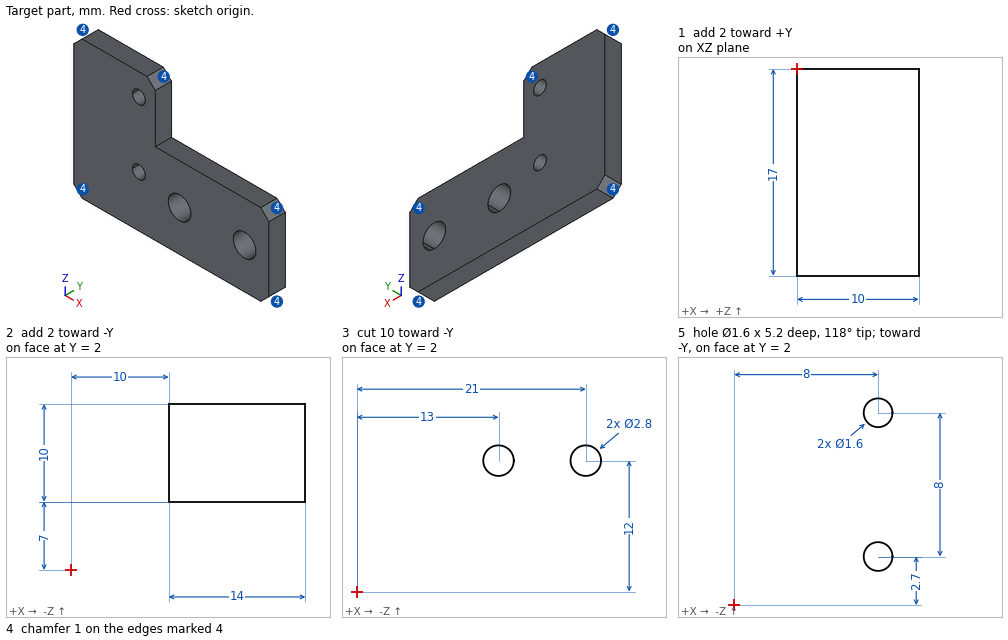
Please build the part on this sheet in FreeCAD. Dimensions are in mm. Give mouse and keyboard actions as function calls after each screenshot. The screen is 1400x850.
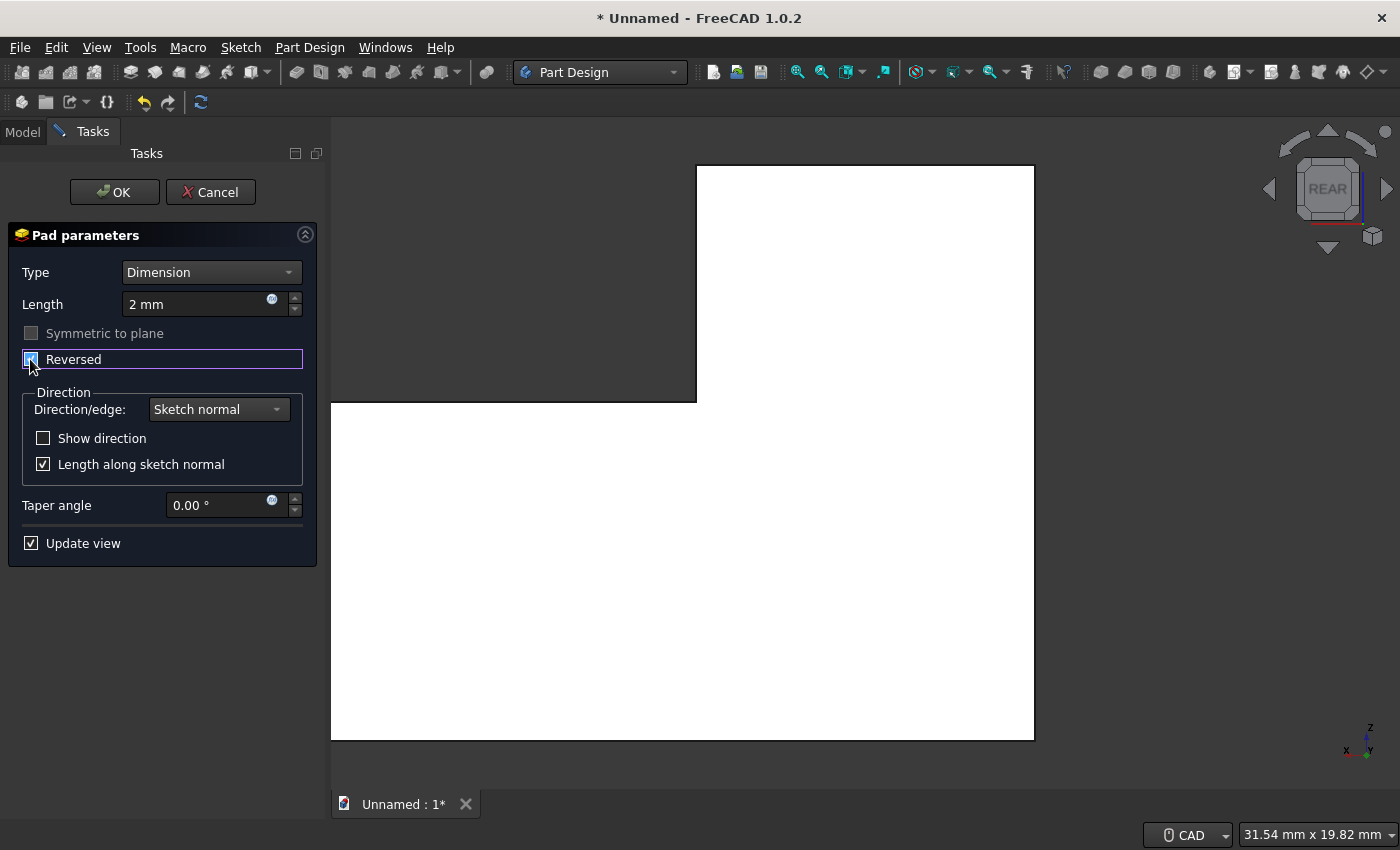
click(115, 192)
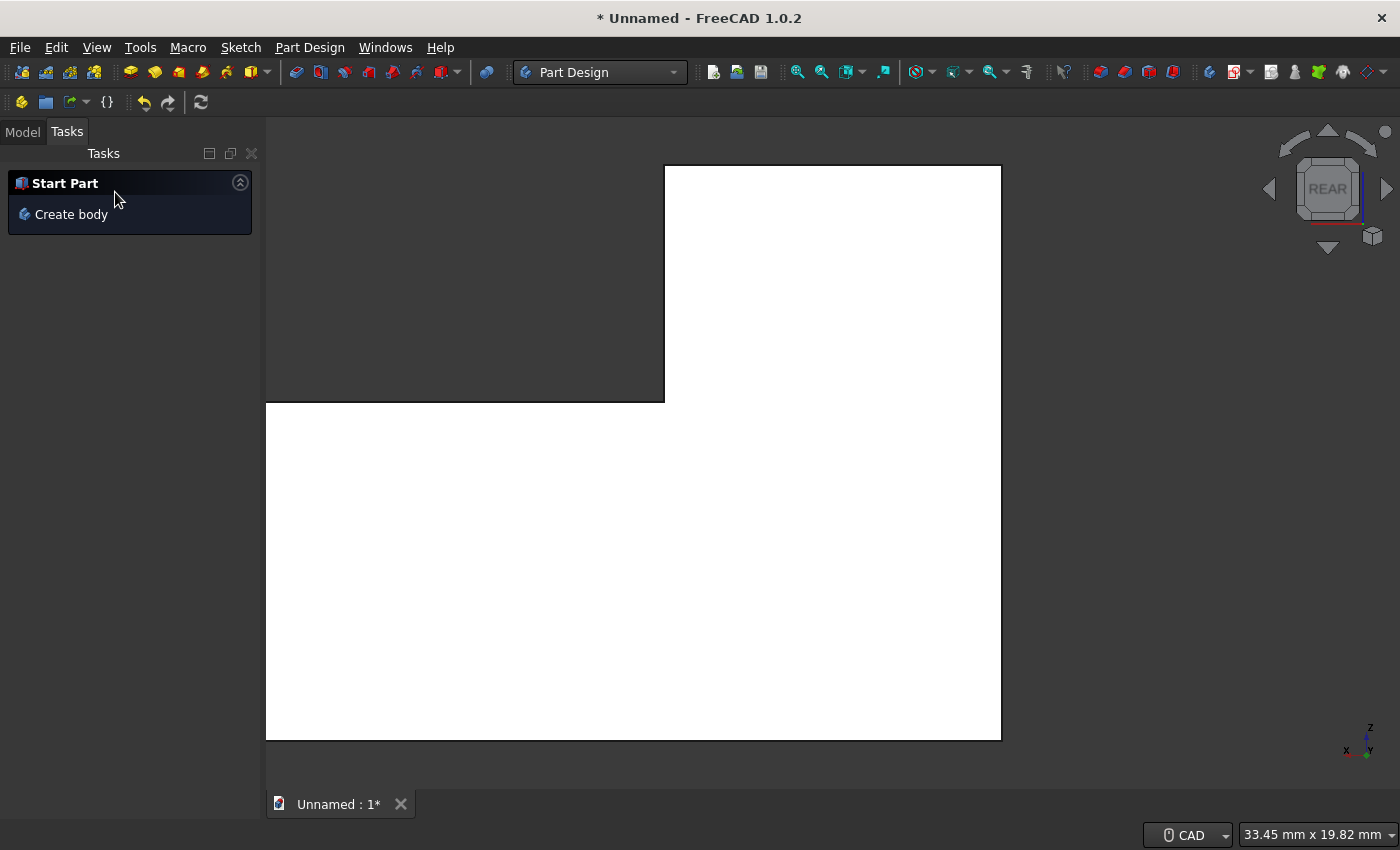
click(798, 72)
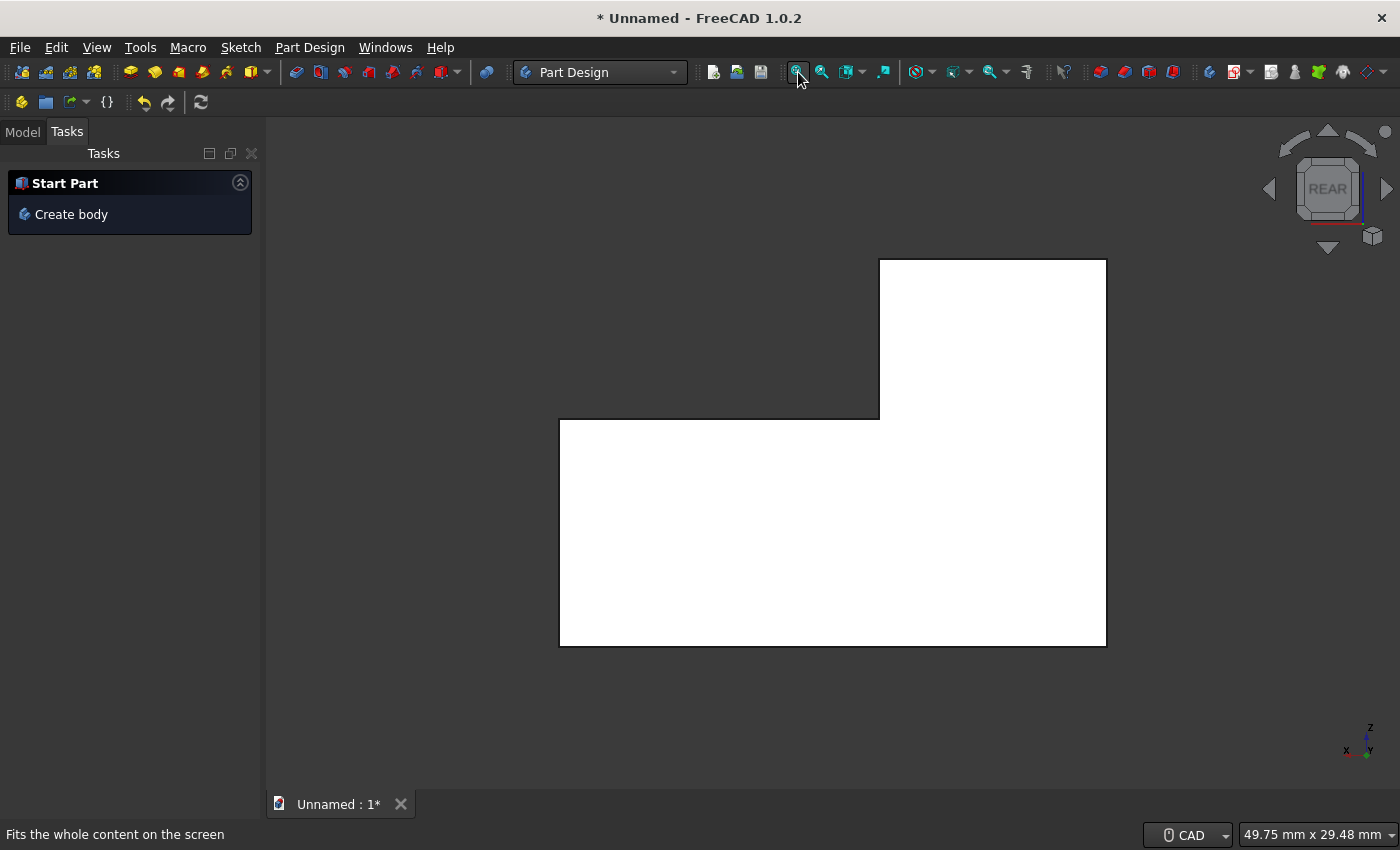
click(989, 507)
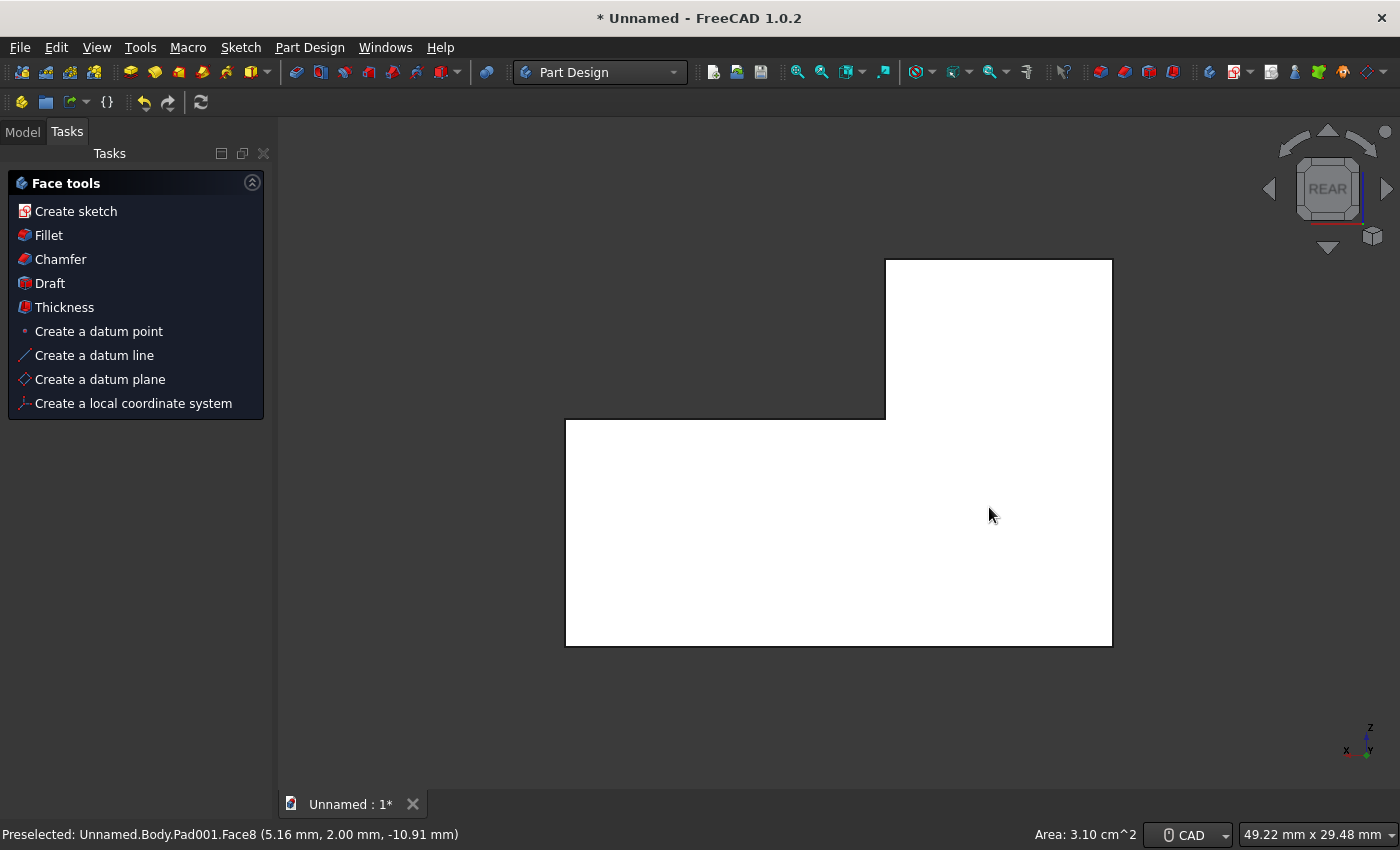
click(1234, 72)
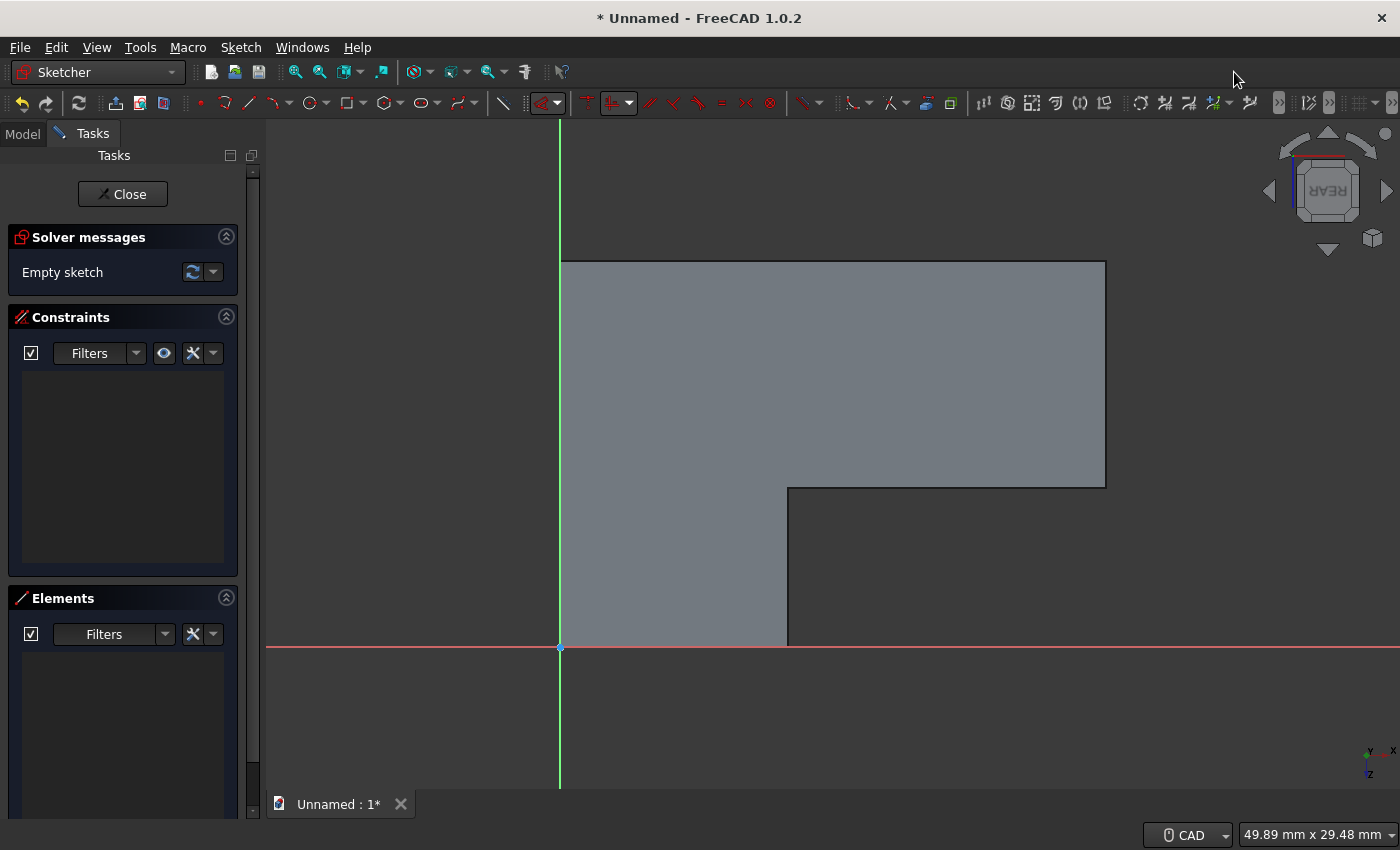
click(310, 104)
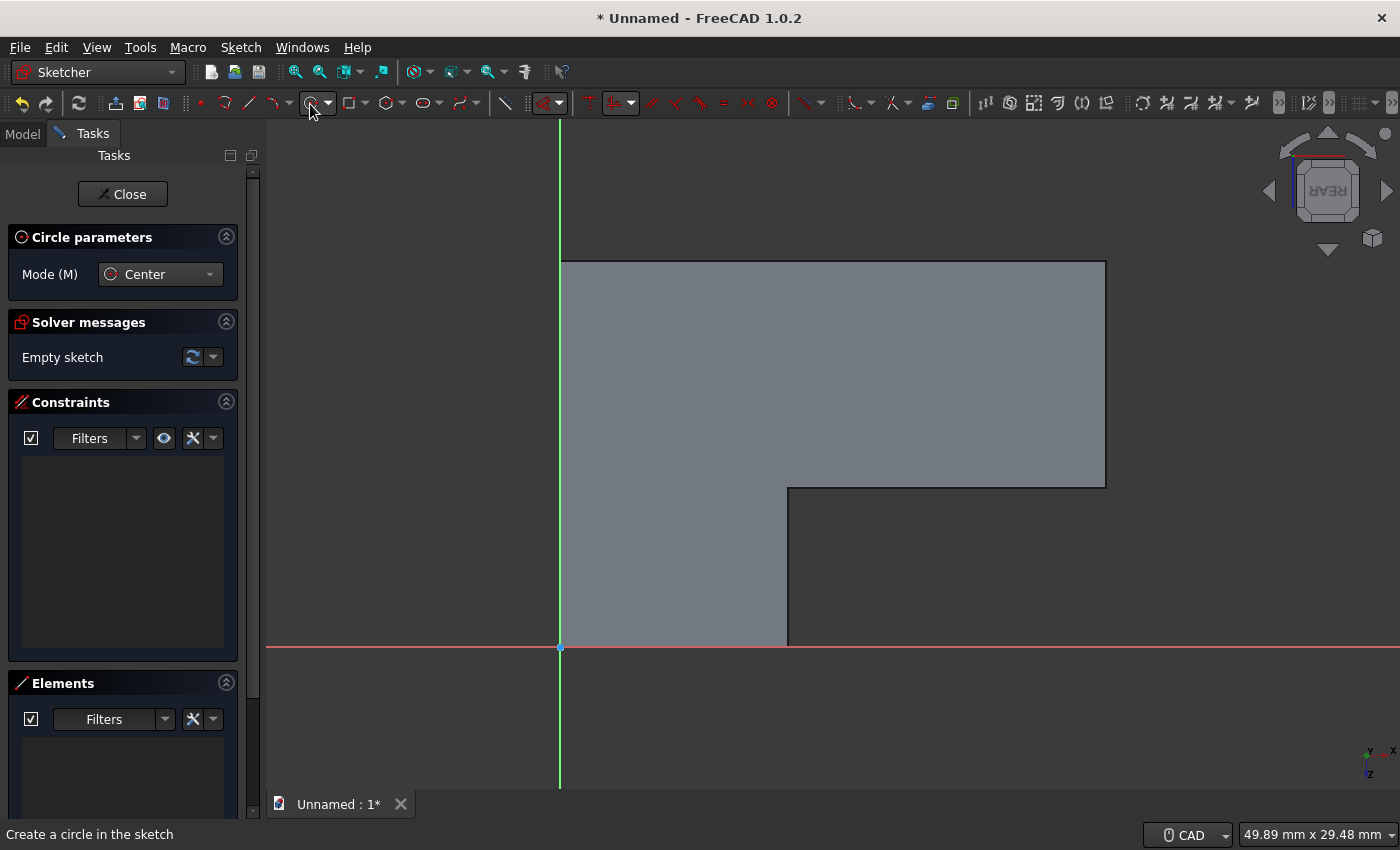
click(1038, 374)
click(1060, 352)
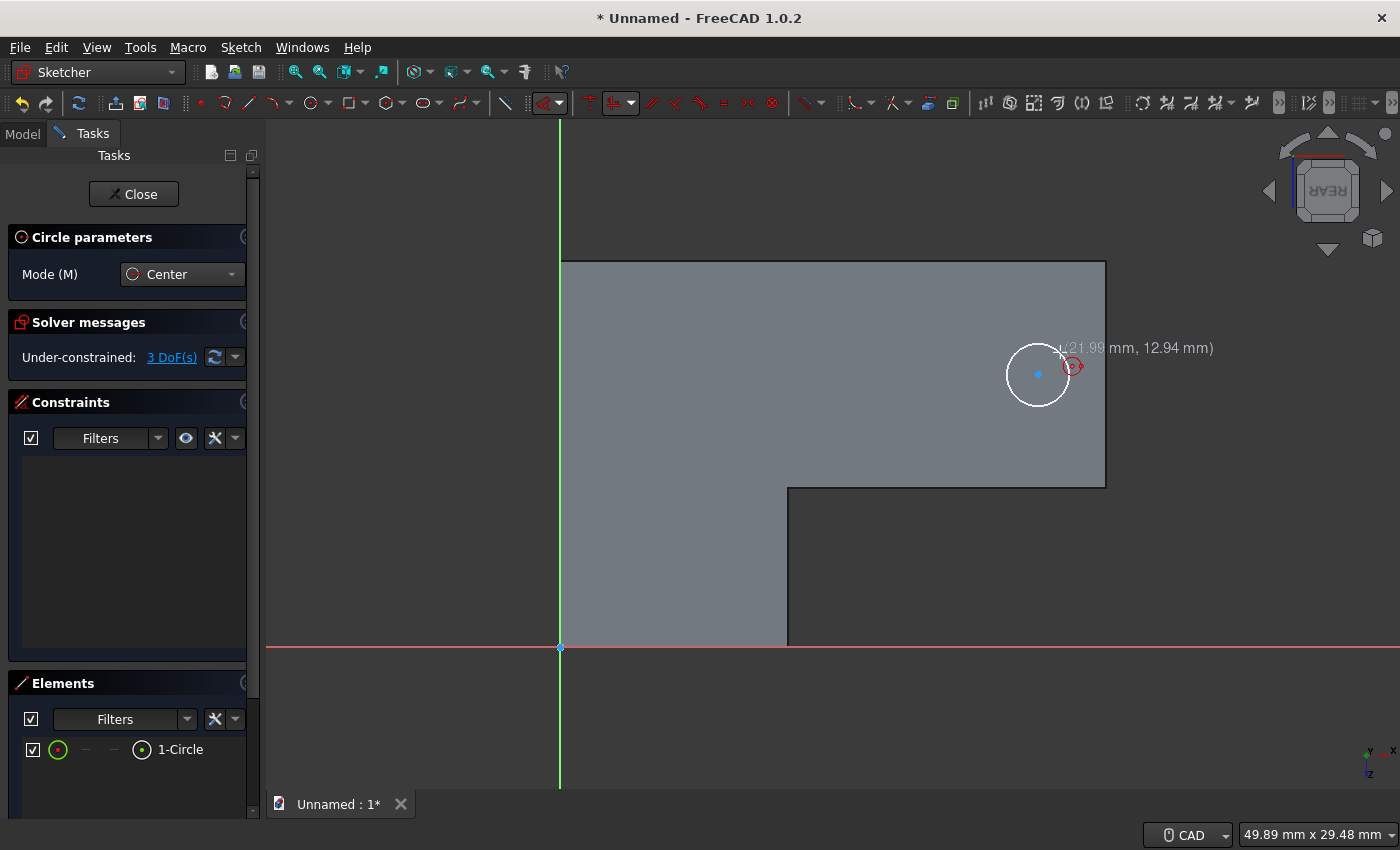
click(856, 374)
click(878, 352)
key(Escape)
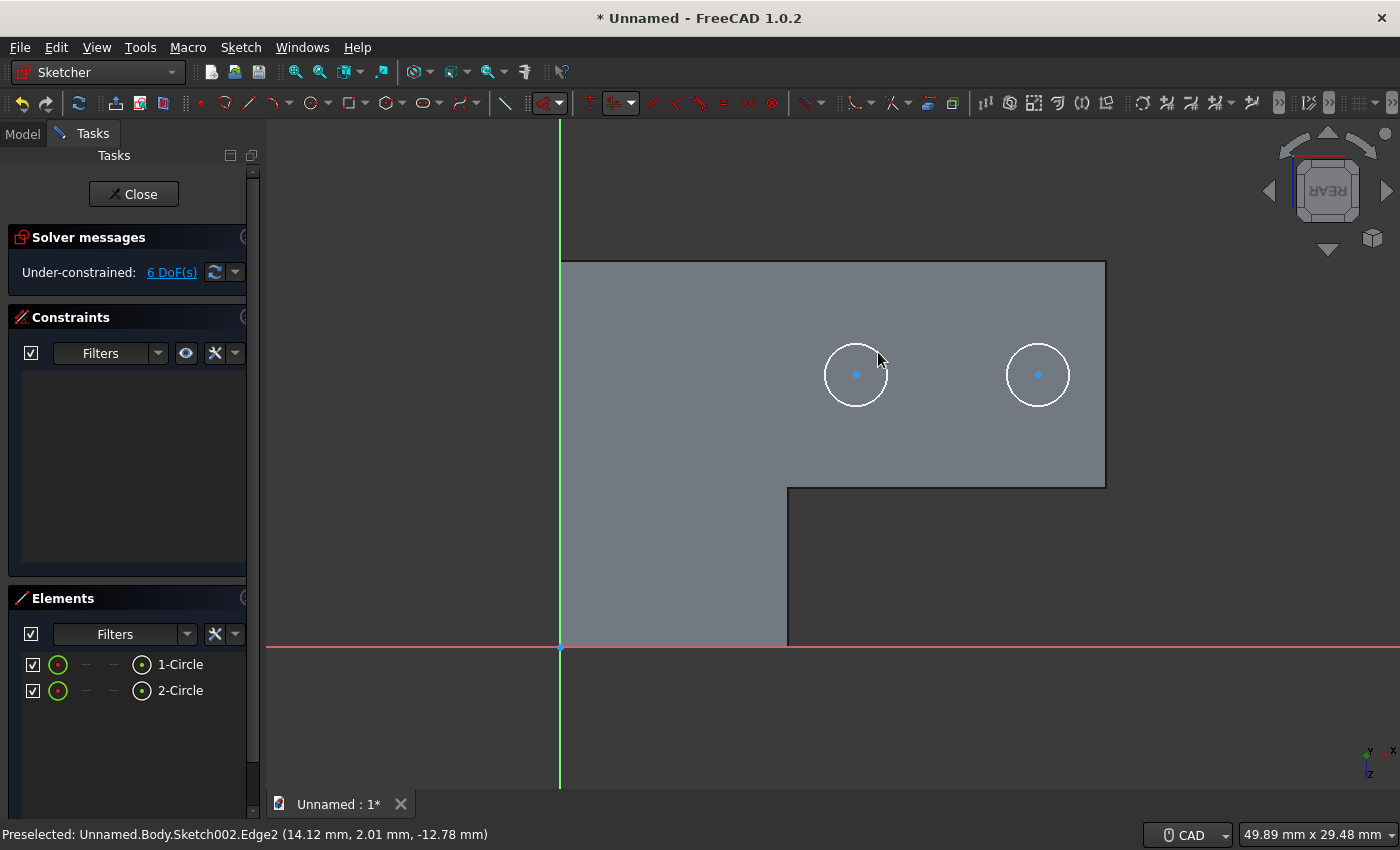
click(1060, 353)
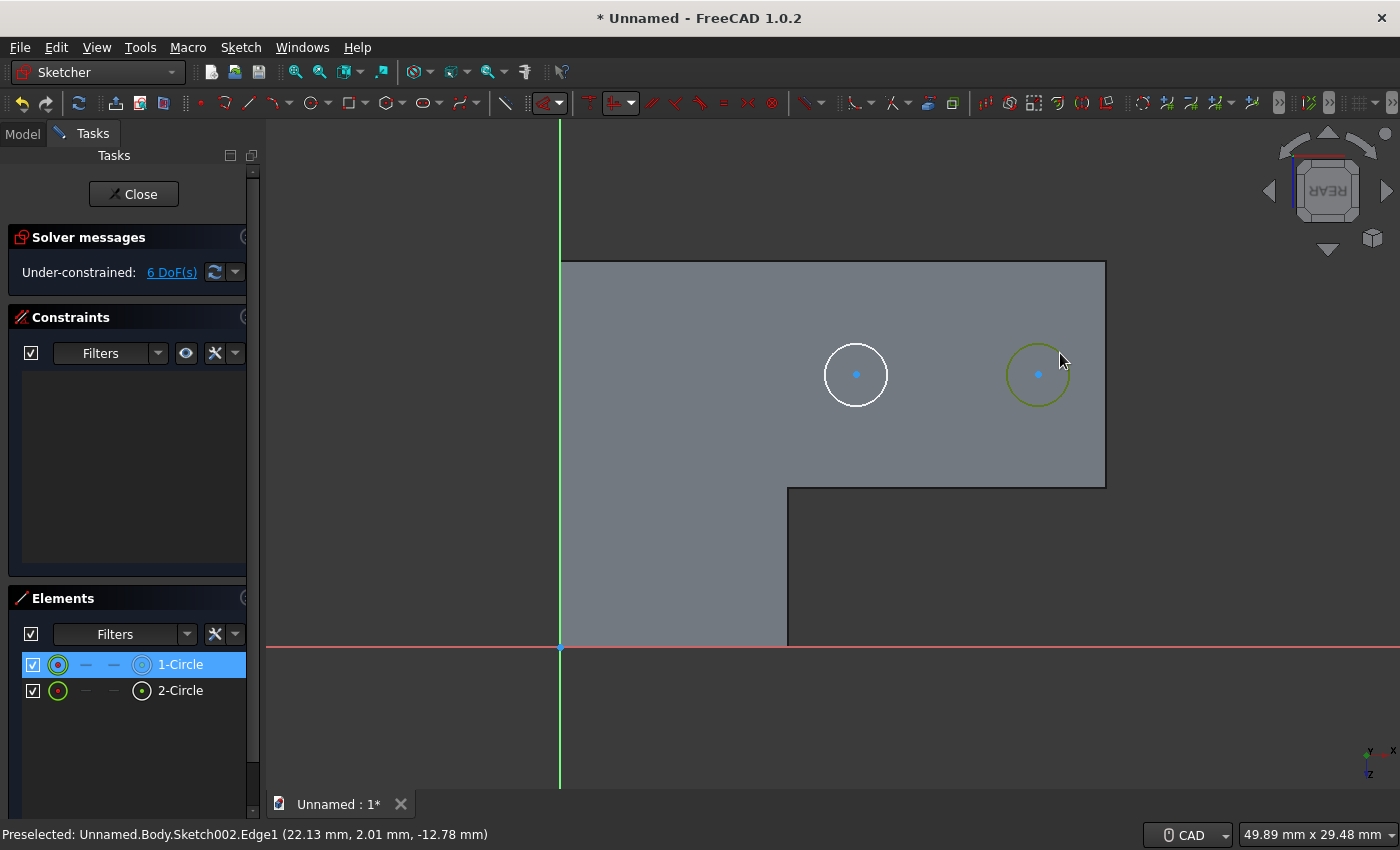
click(878, 353)